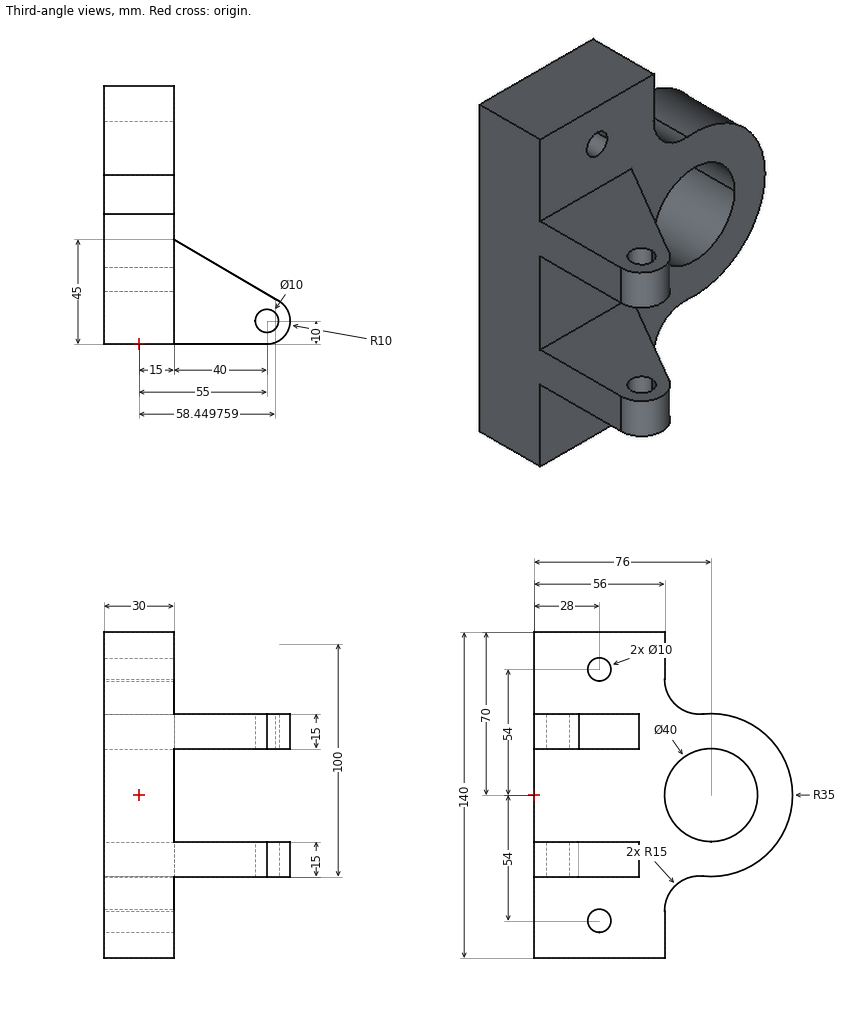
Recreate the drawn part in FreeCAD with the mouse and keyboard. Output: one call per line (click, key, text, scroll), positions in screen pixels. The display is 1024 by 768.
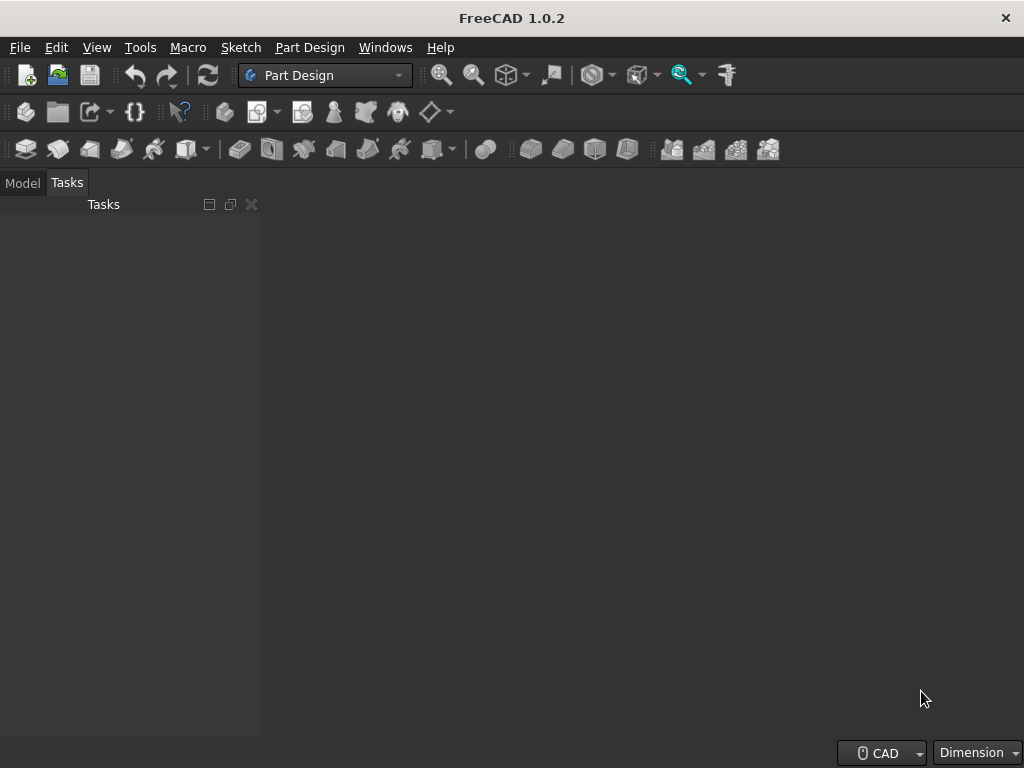
key(ctrl+n)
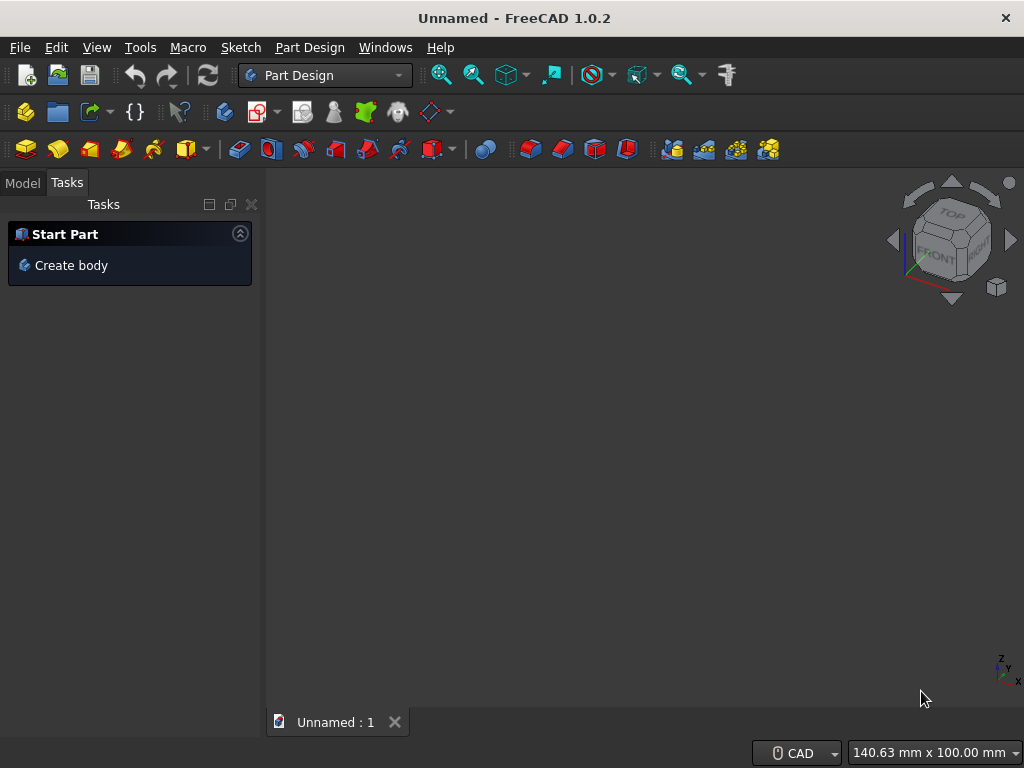
click(258, 112)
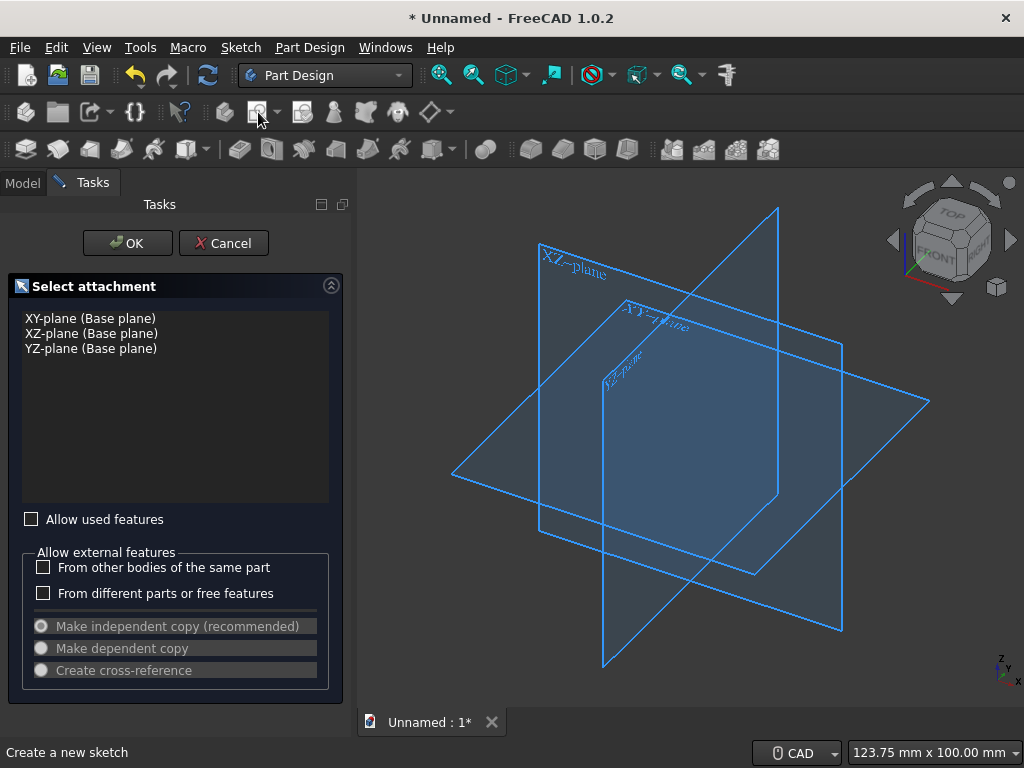
click(82, 348)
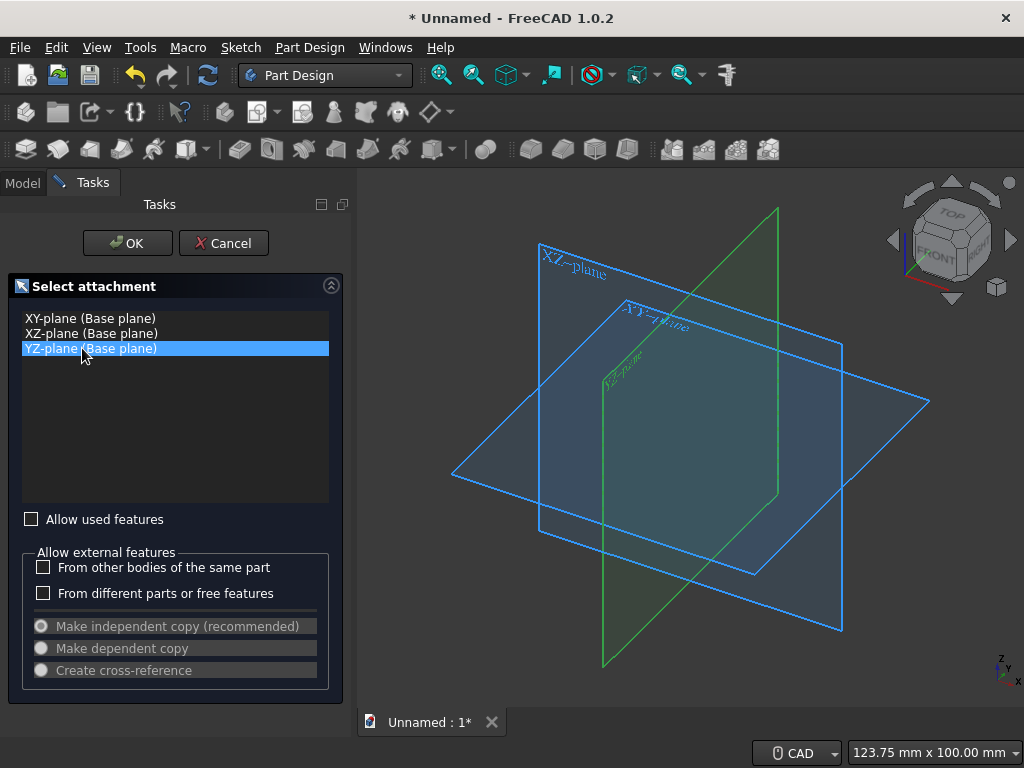
click(128, 243)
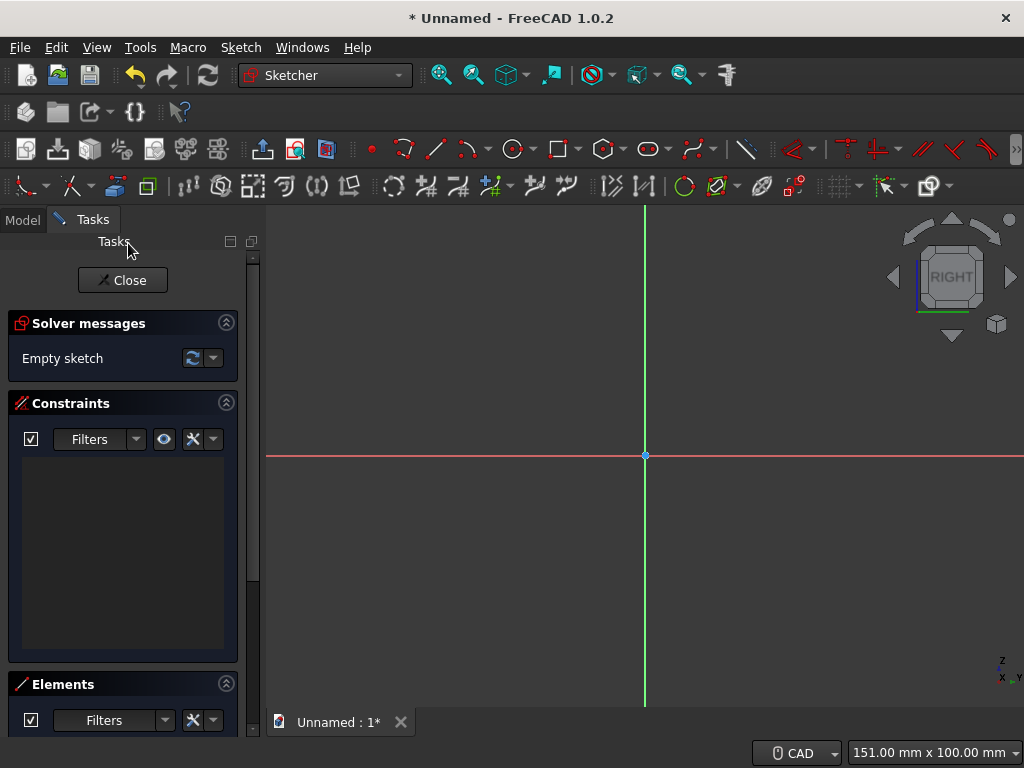
scroll(294, 456, down, 4)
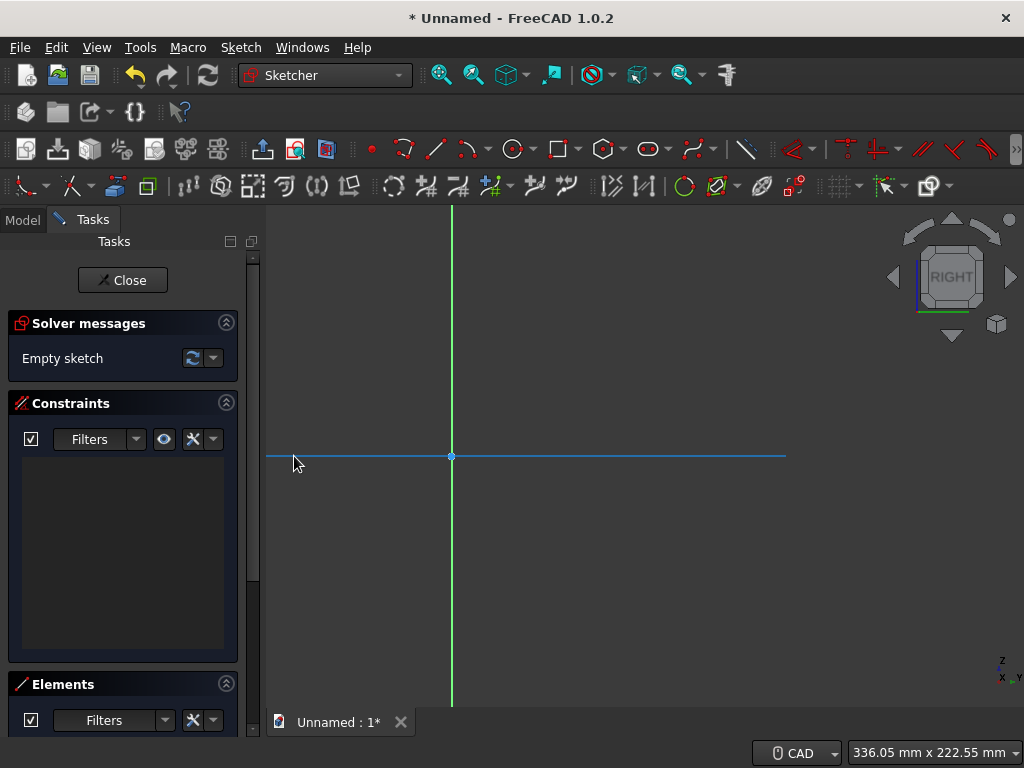
key(g)
key(m)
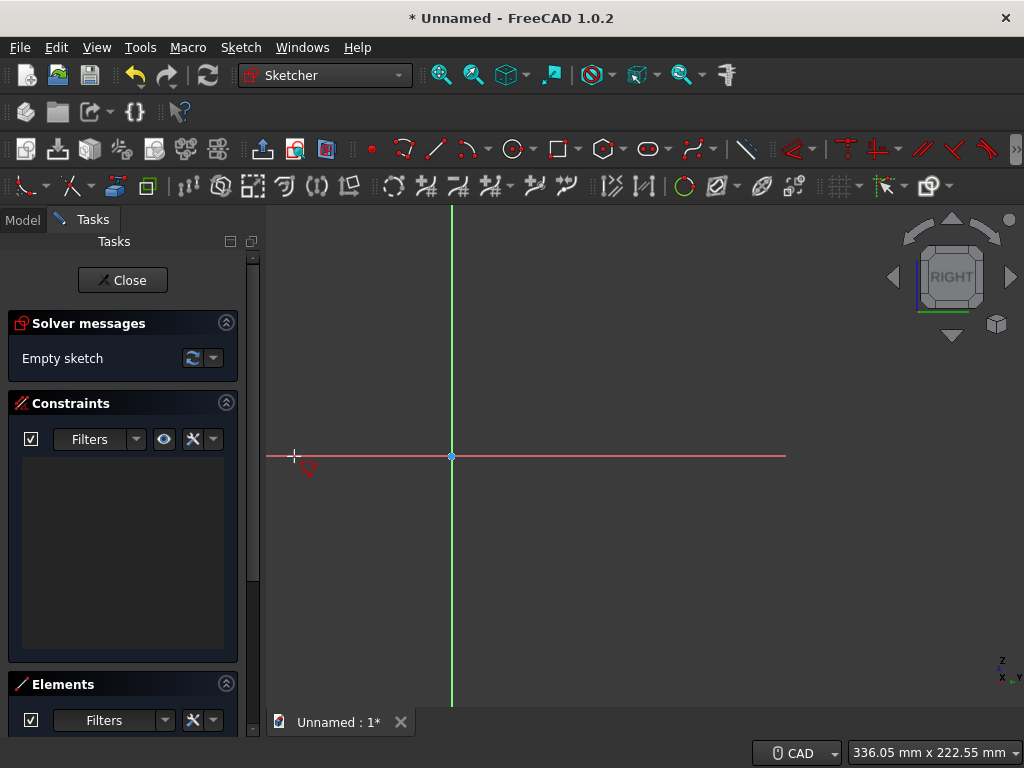
click(578, 344)
click(578, 298)
click(452, 298)
click(461, 614)
click(578, 614)
click(578, 568)
right_click(578, 568)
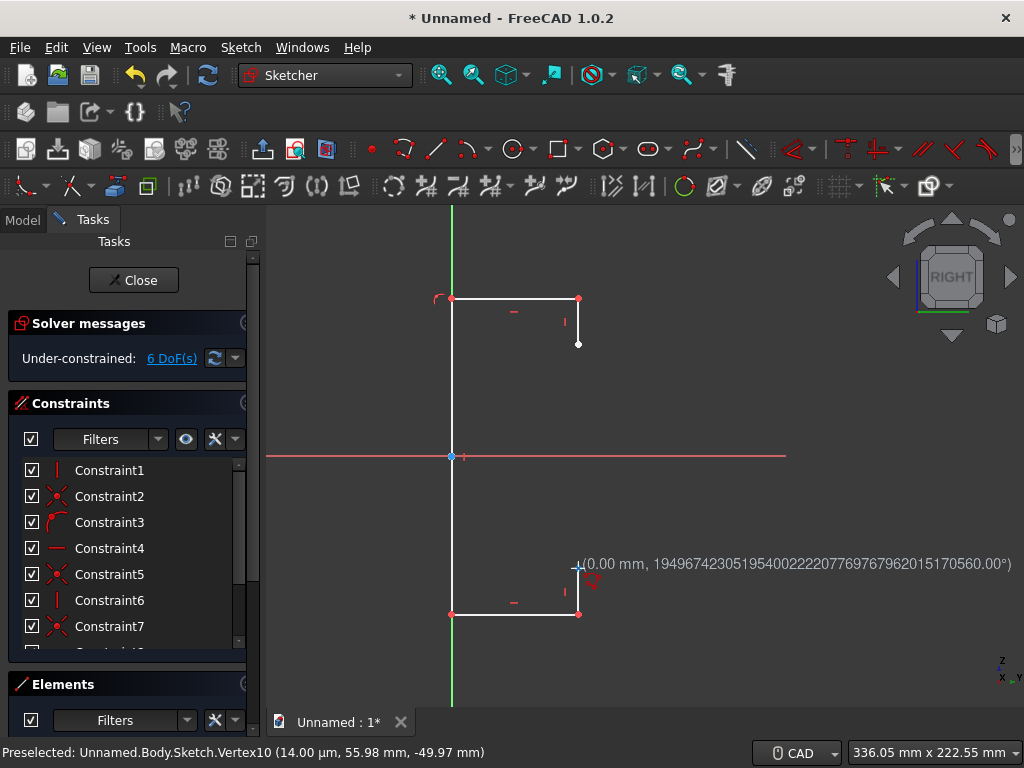
key(g)
key(3)
key(a)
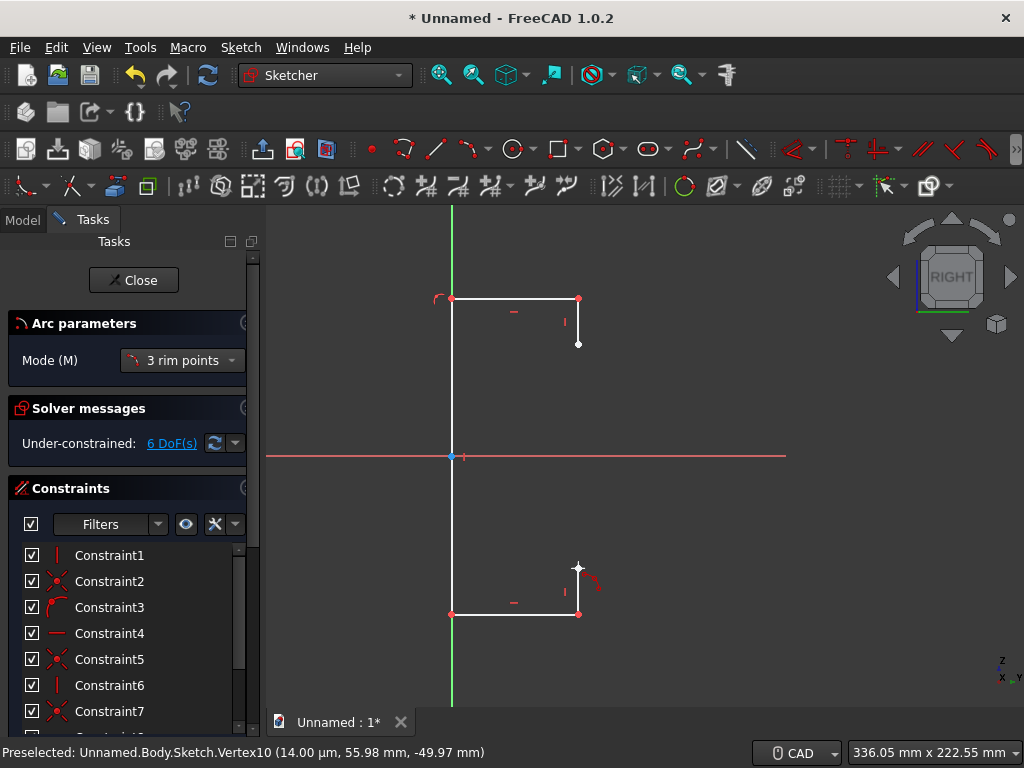
click(578, 569)
click(615, 535)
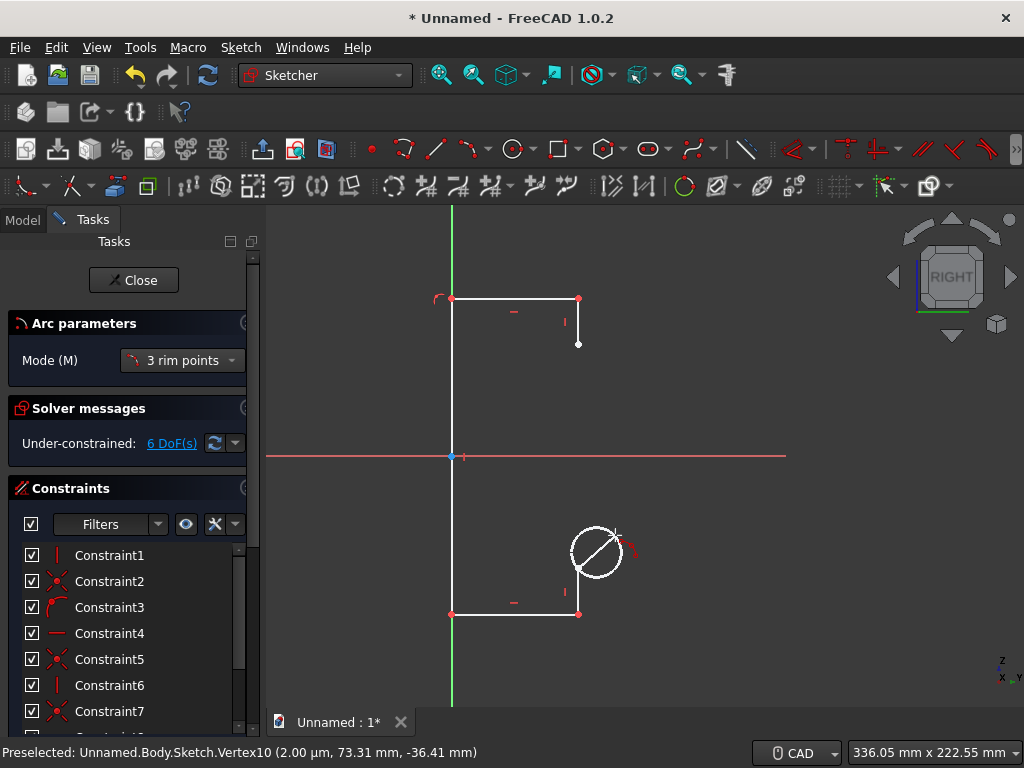
scroll(589, 543, up, 2)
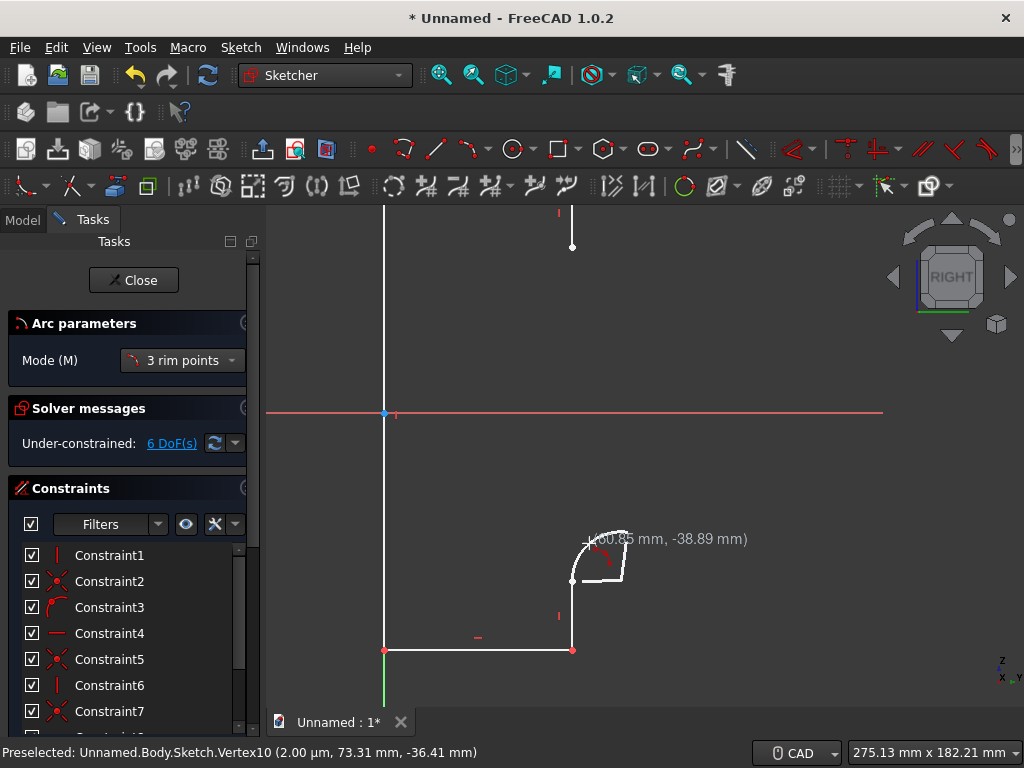
click(589, 543)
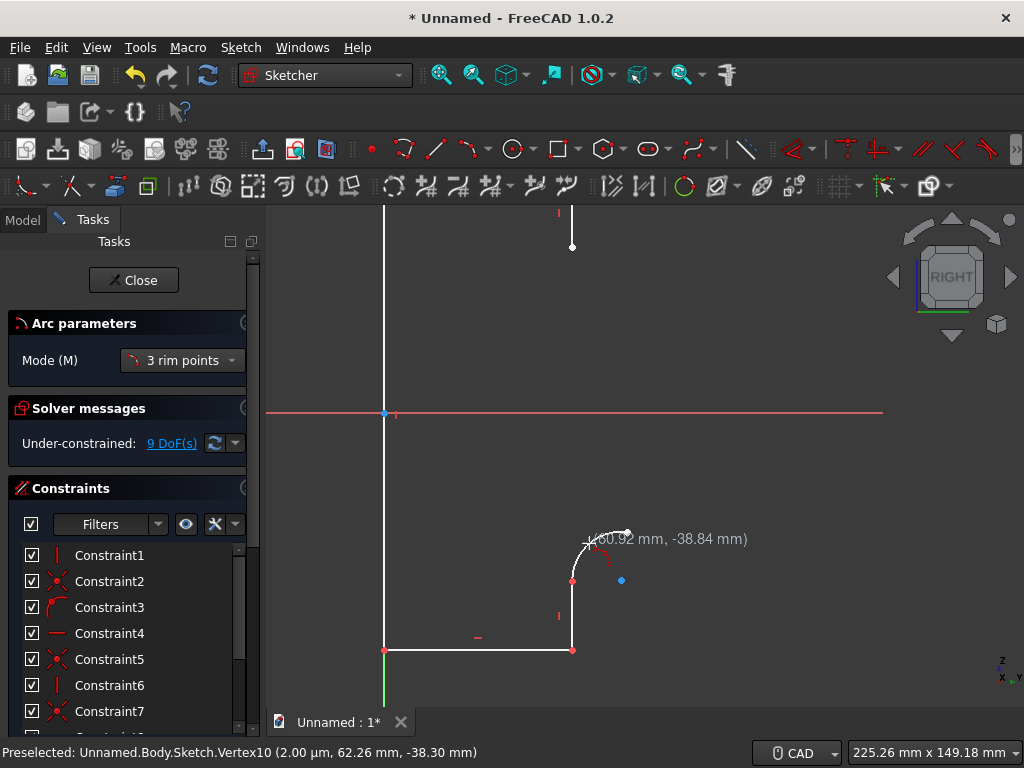
click(628, 532)
click(628, 296)
click(751, 452)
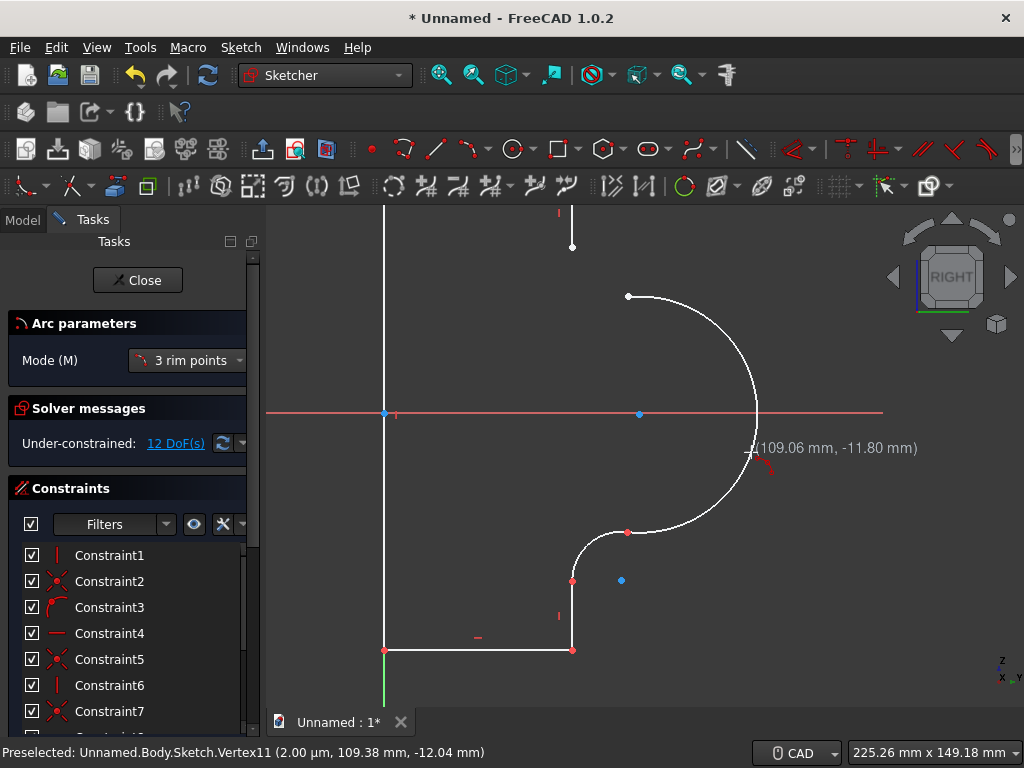
click(628, 297)
click(572, 247)
click(589, 283)
key(Escape)